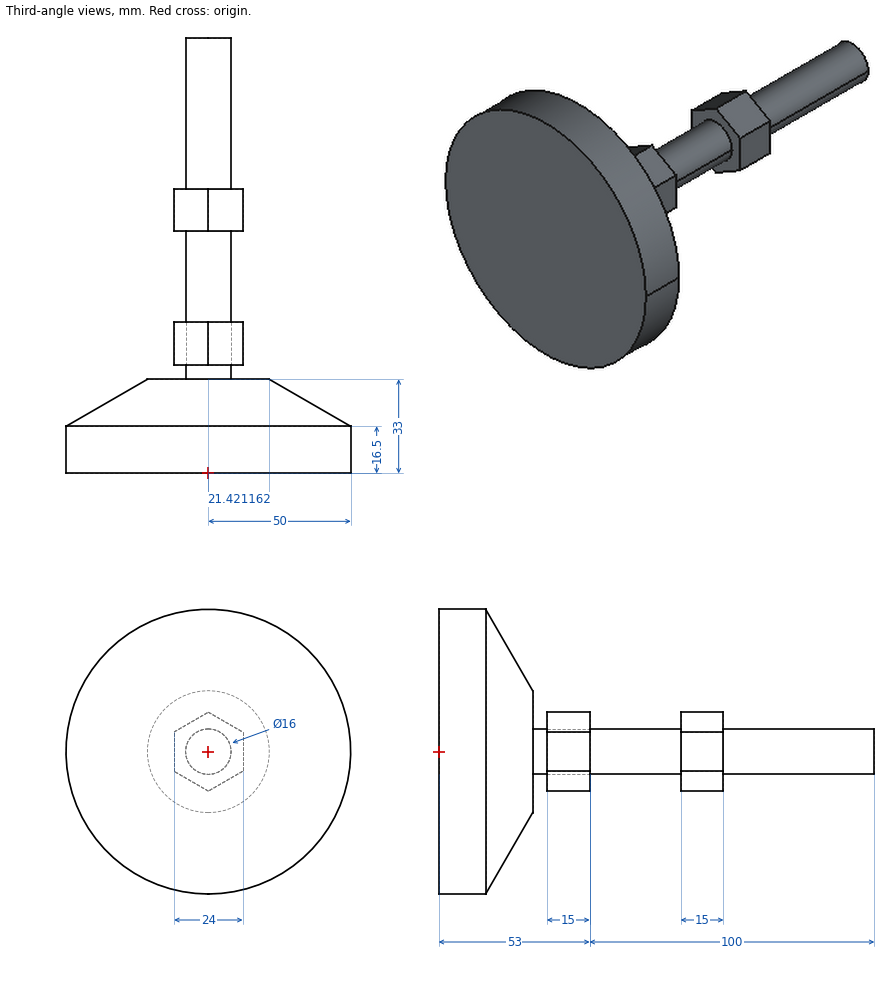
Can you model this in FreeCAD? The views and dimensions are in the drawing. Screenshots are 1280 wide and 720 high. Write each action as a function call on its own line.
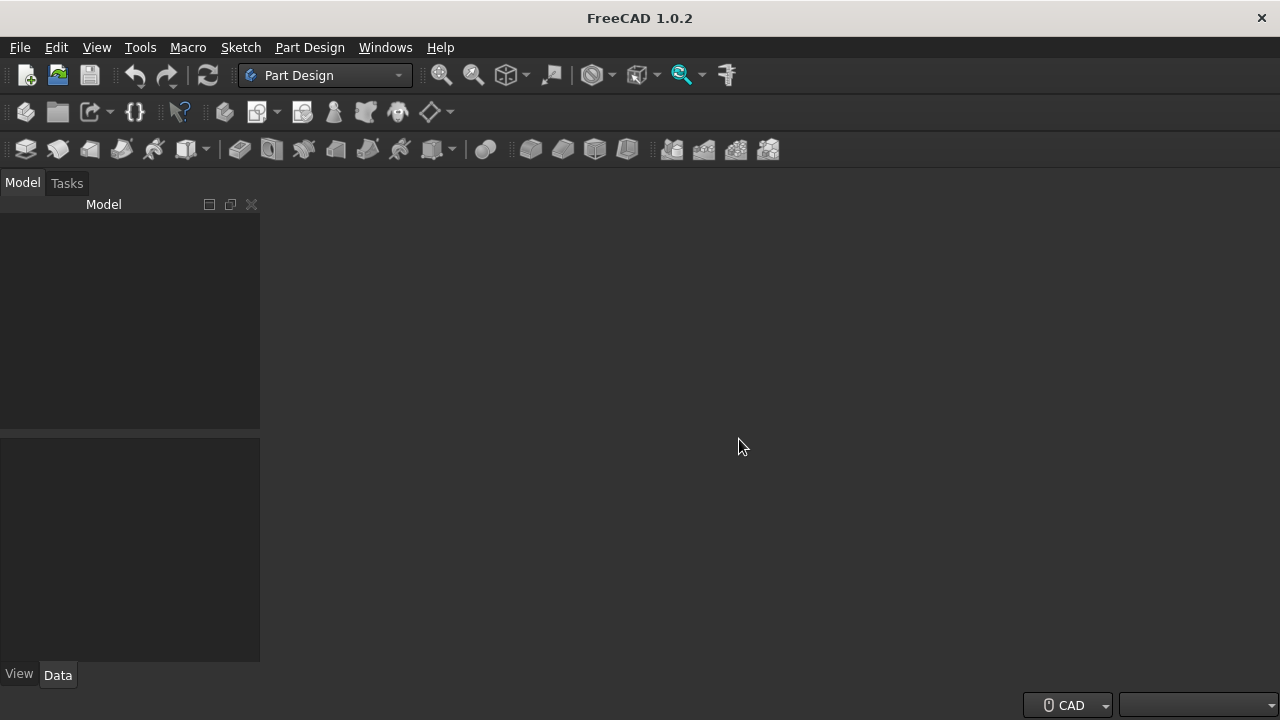
click(26, 76)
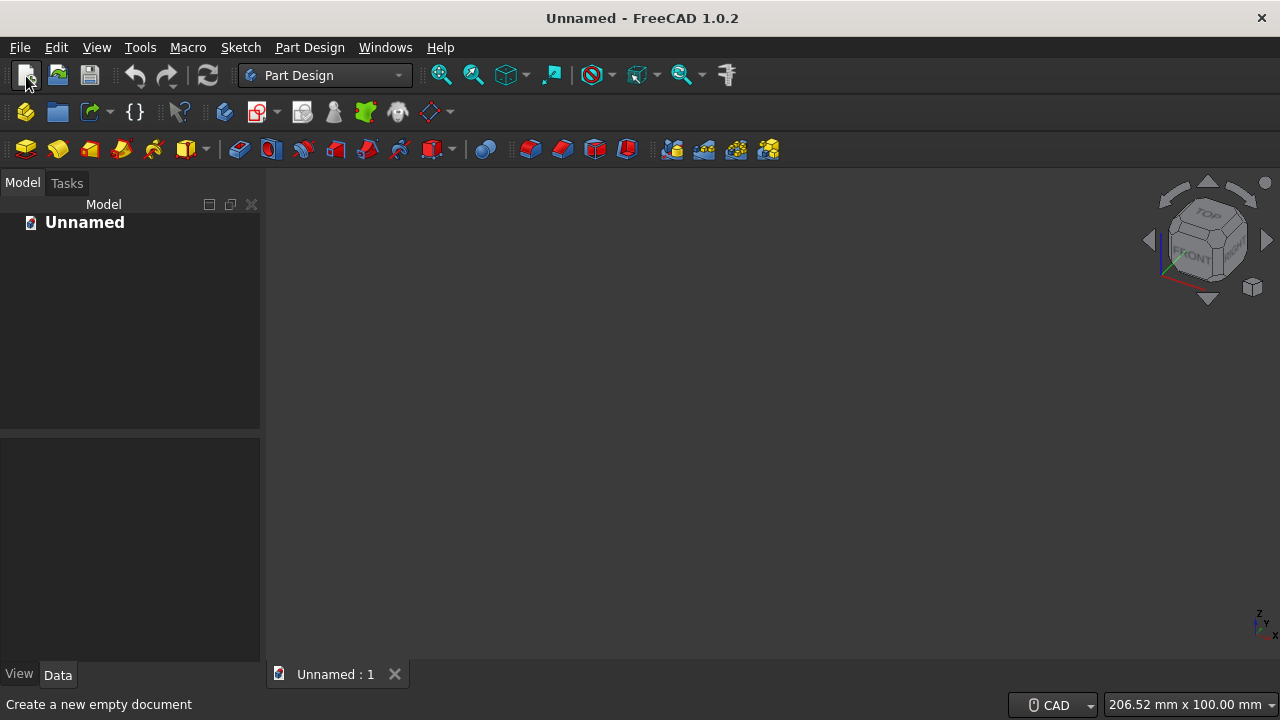
click(258, 112)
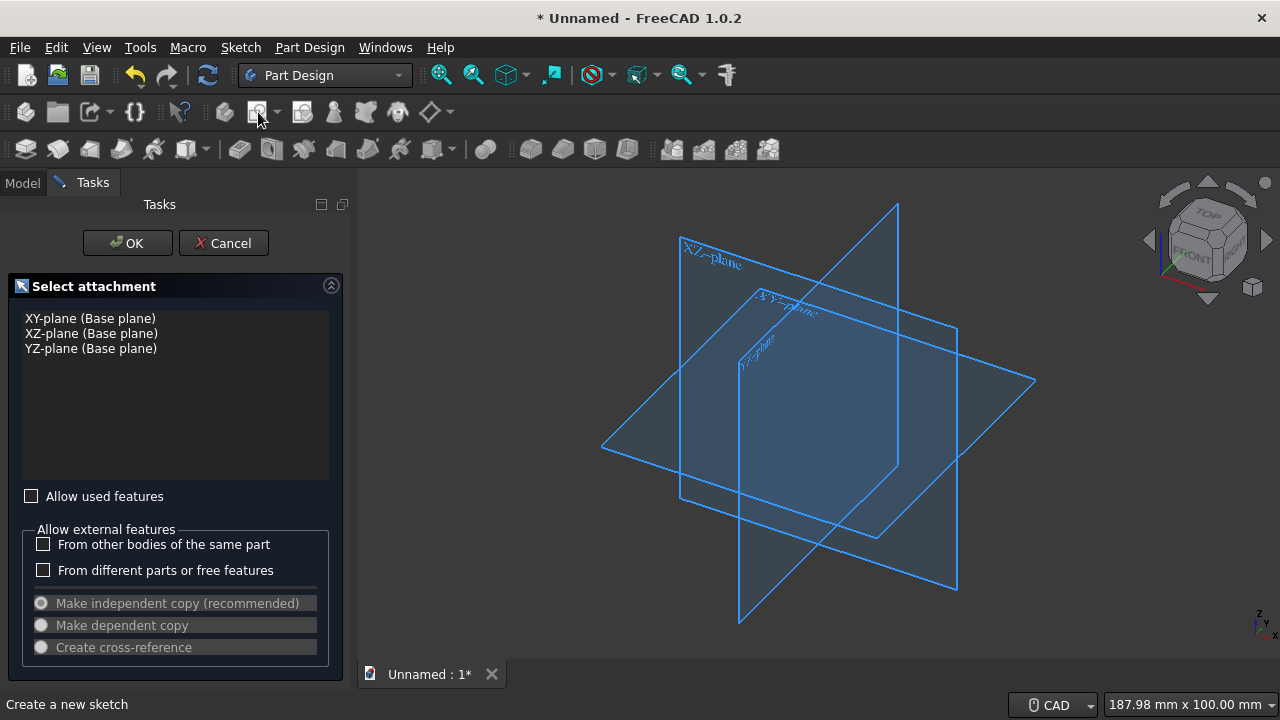
click(82, 318)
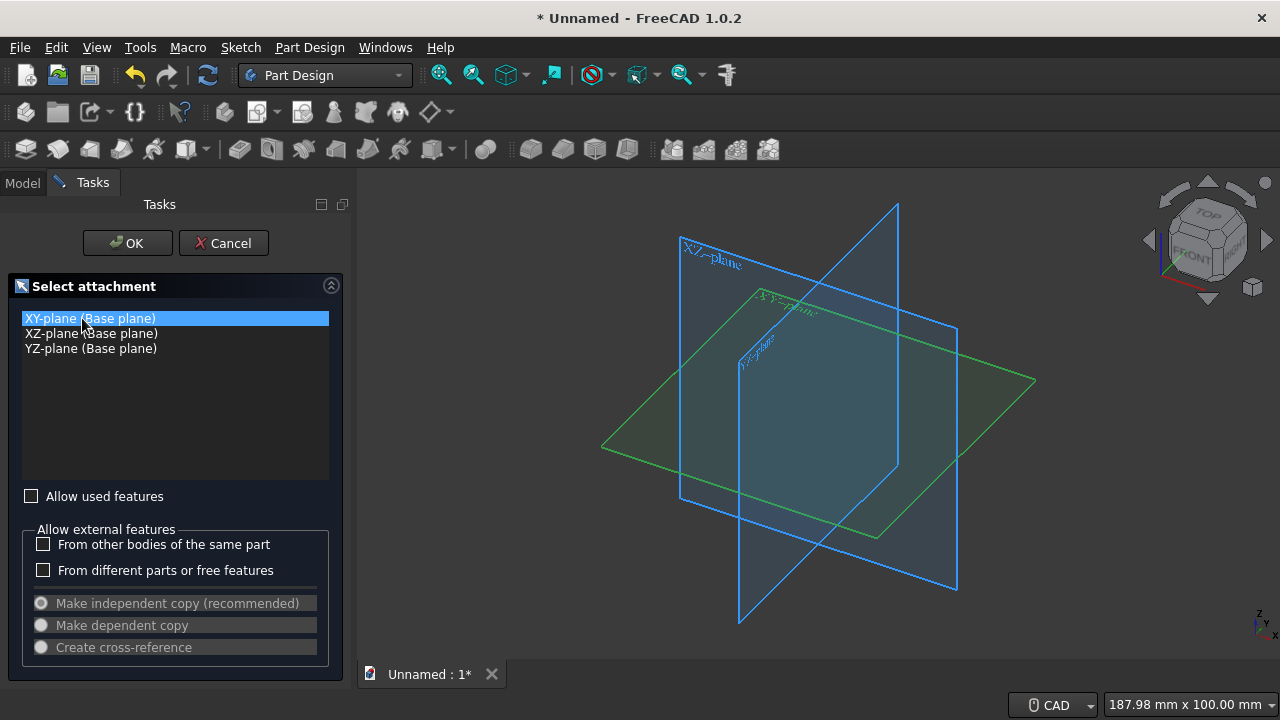
click(128, 243)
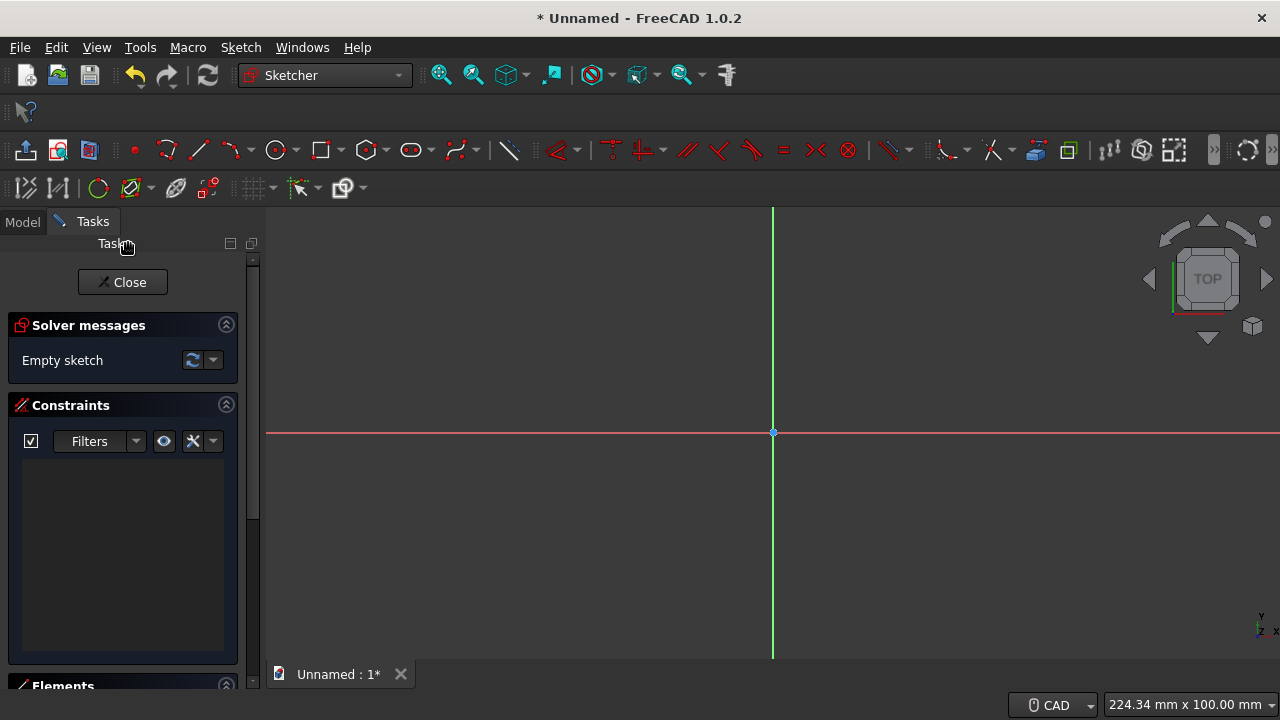
scroll(1107, 268, up, 3)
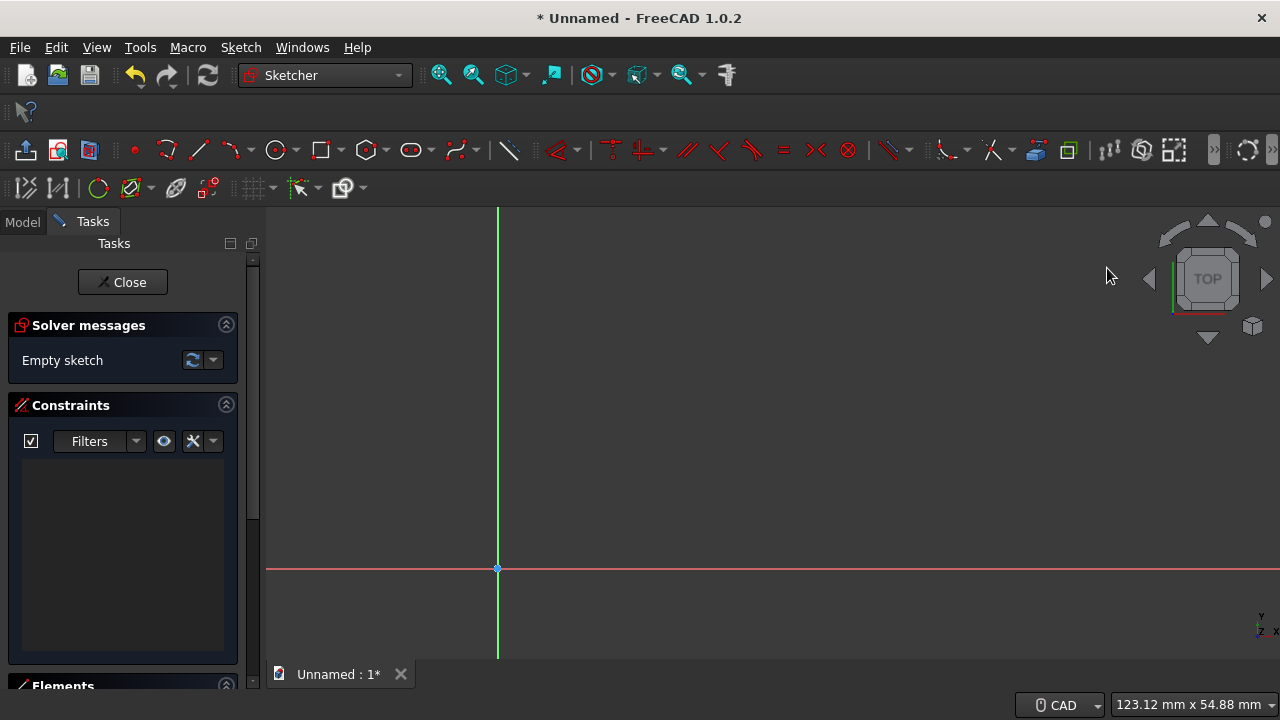
click(168, 150)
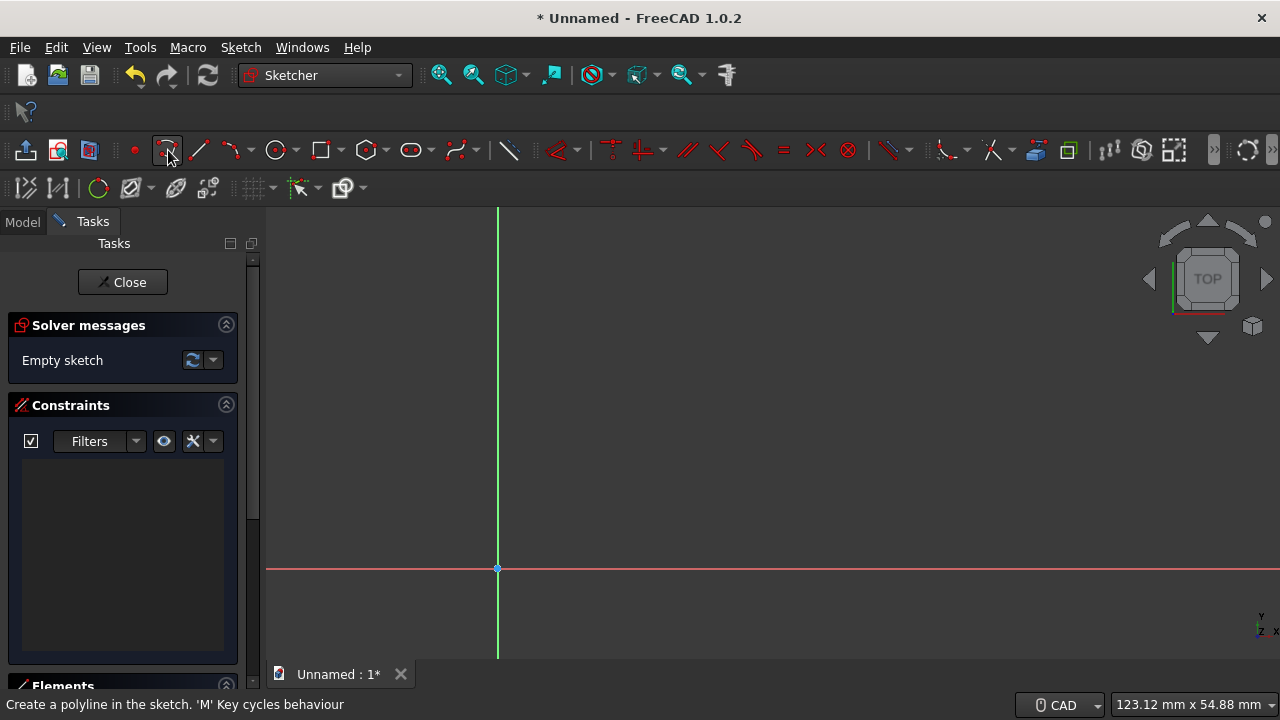
click(498, 569)
click(910, 560)
click(910, 433)
click(674, 297)
click(507, 297)
click(498, 569)
key(Escape)
key(Escape)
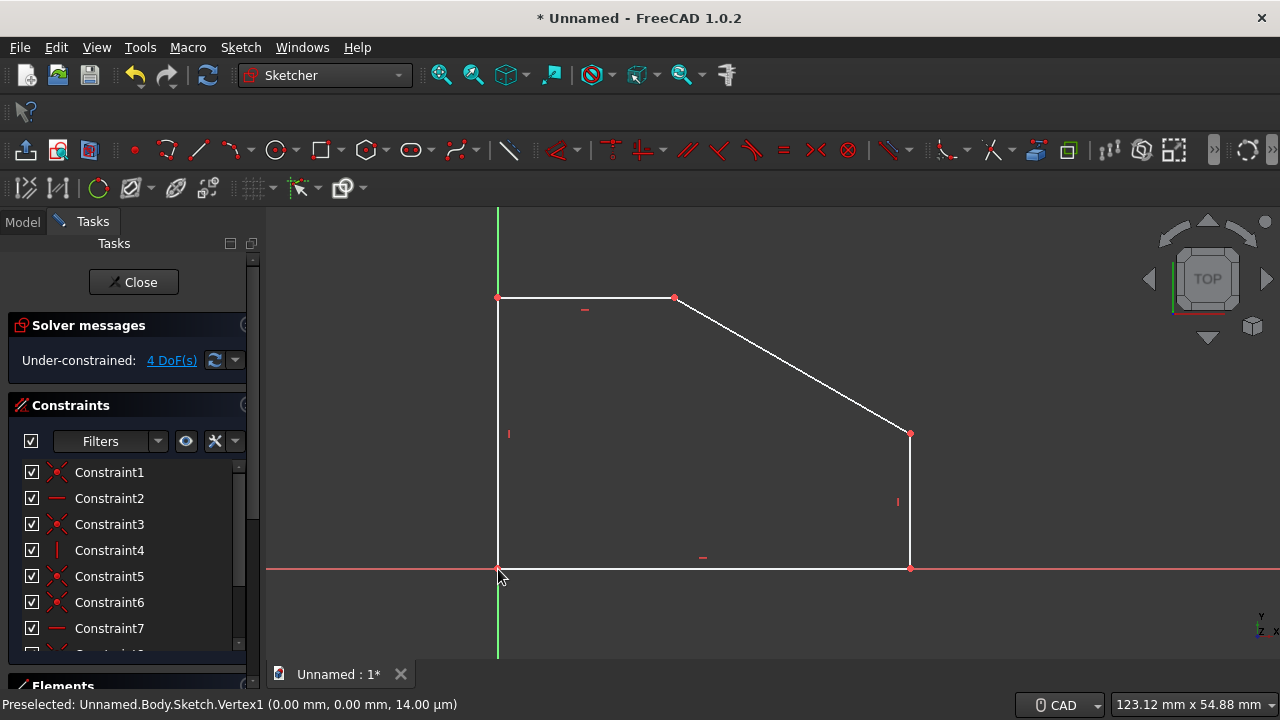
click(621, 569)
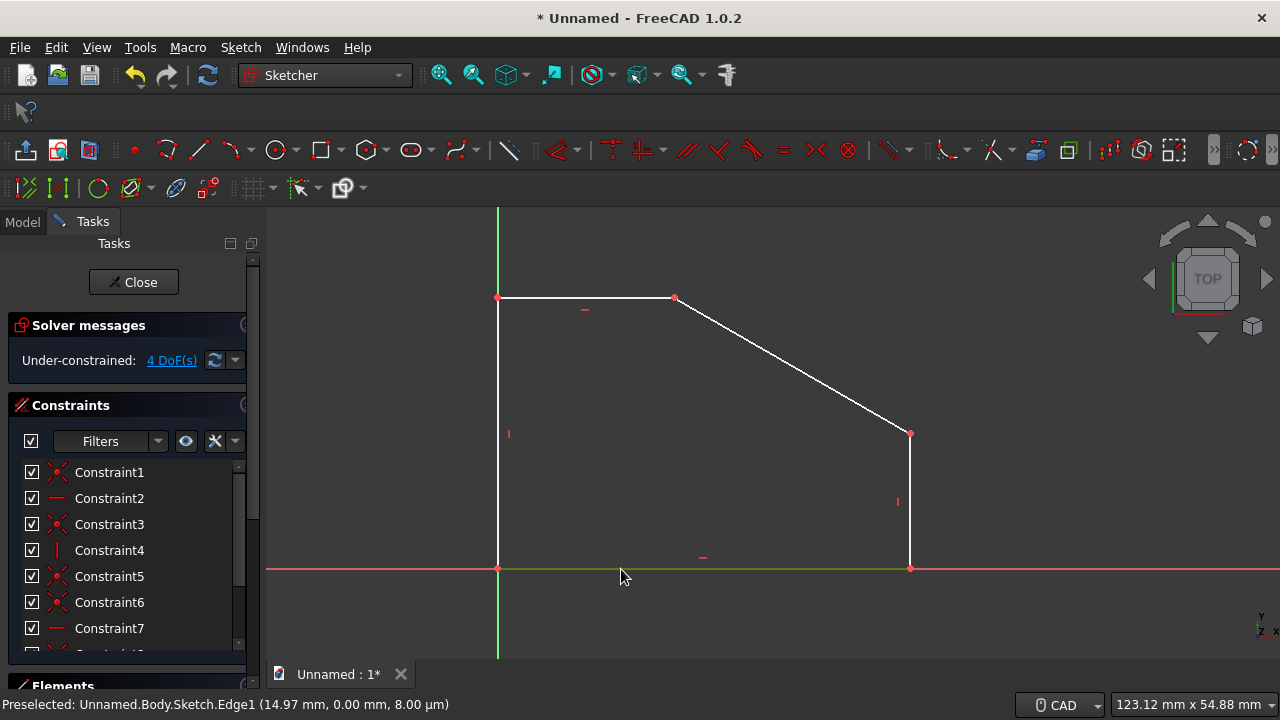
click(580, 150)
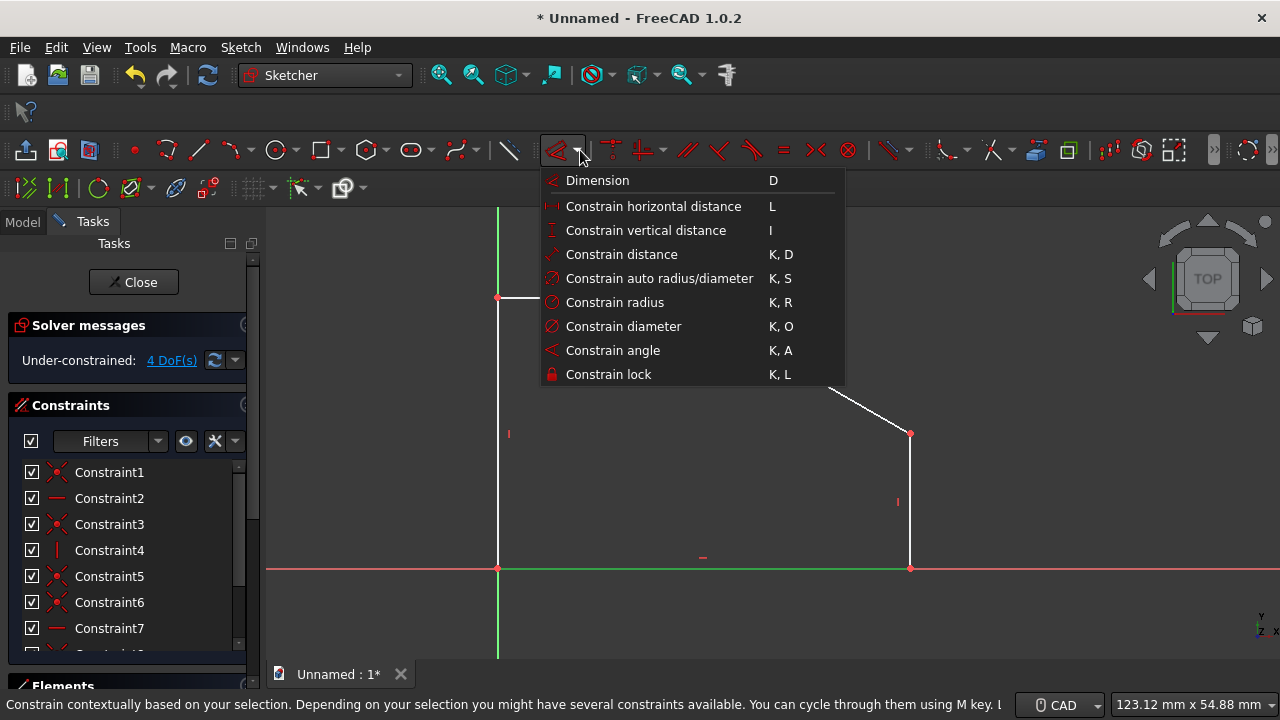
click(693, 206)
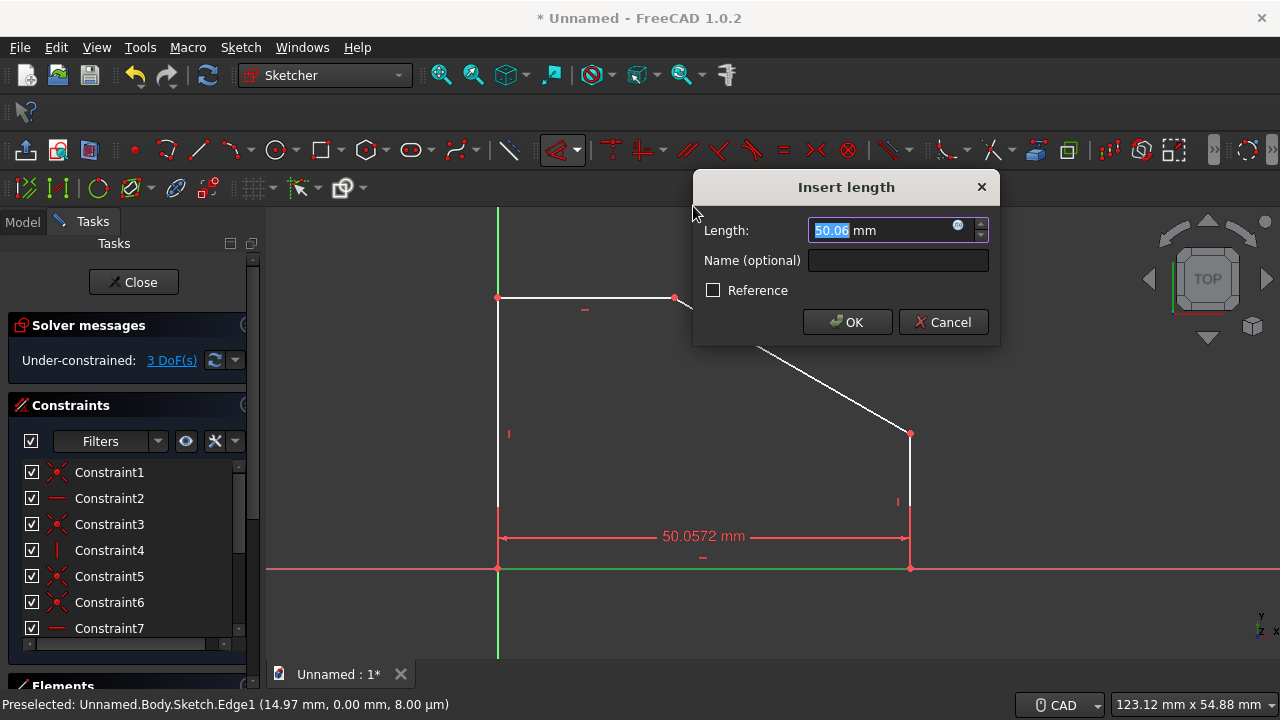
text(50)
key(Return)